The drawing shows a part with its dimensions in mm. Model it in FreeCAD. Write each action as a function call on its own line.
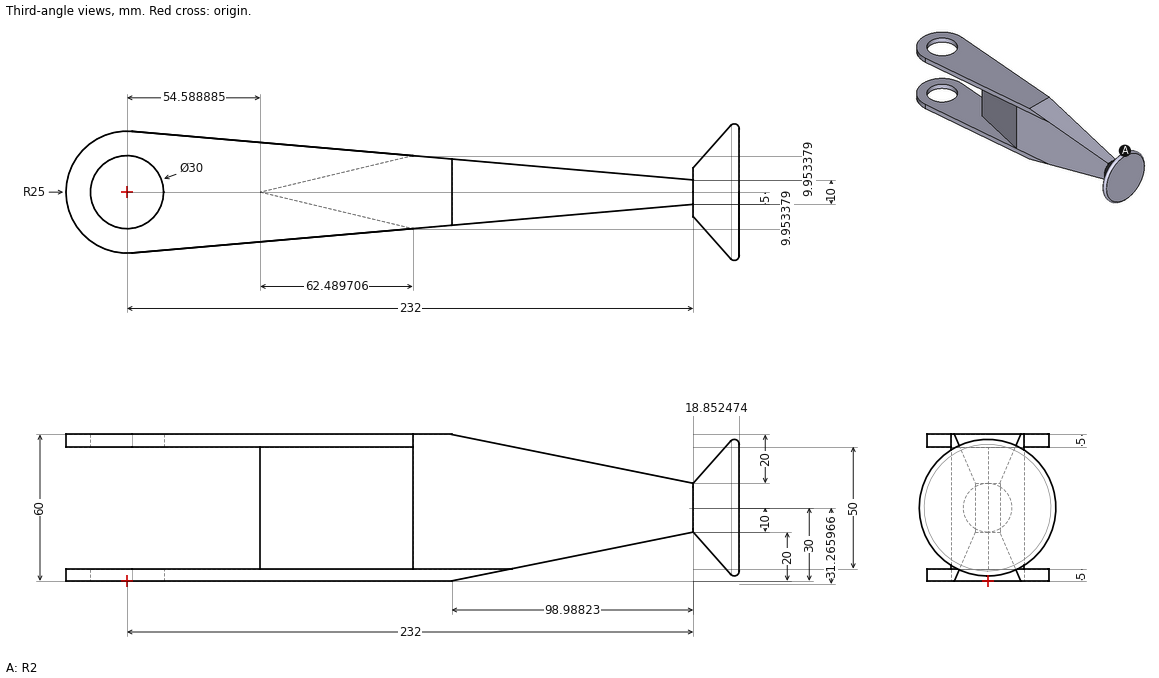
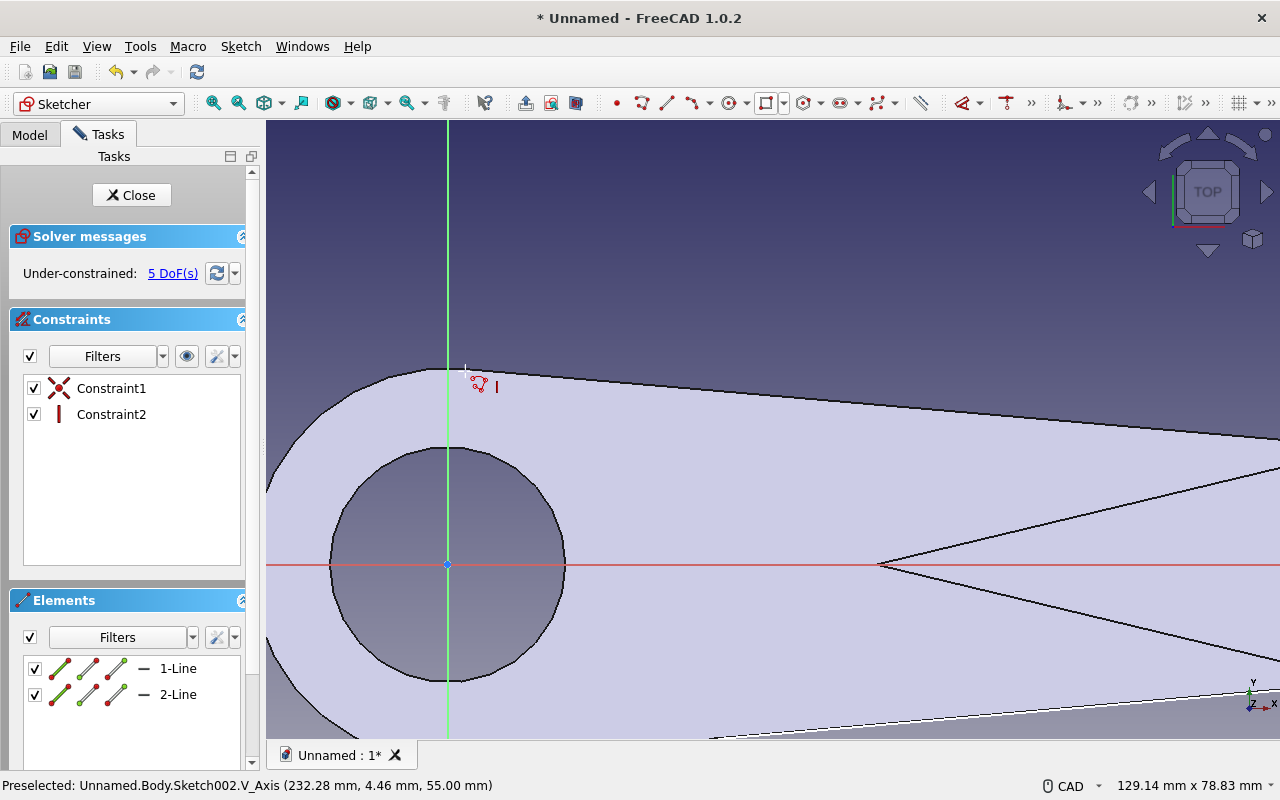
click(465, 369)
right_click(465, 369)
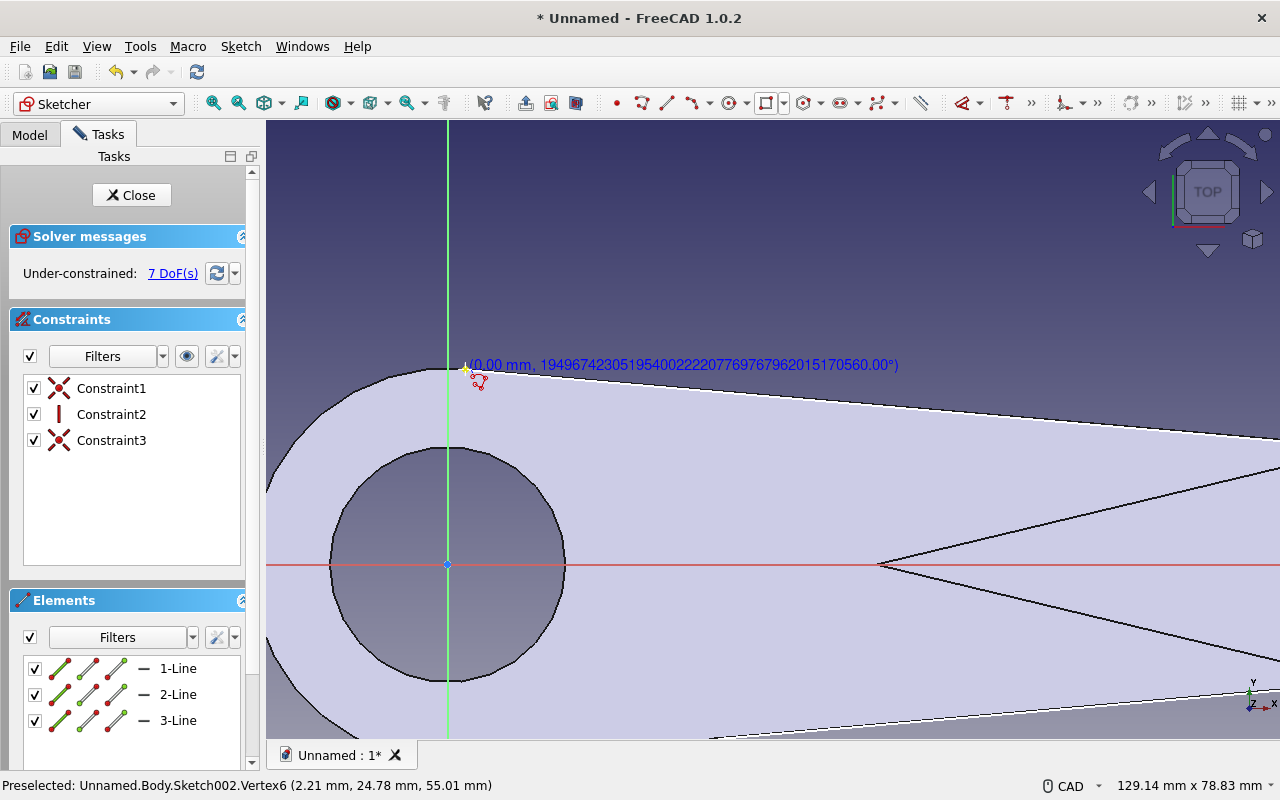
click(692, 104)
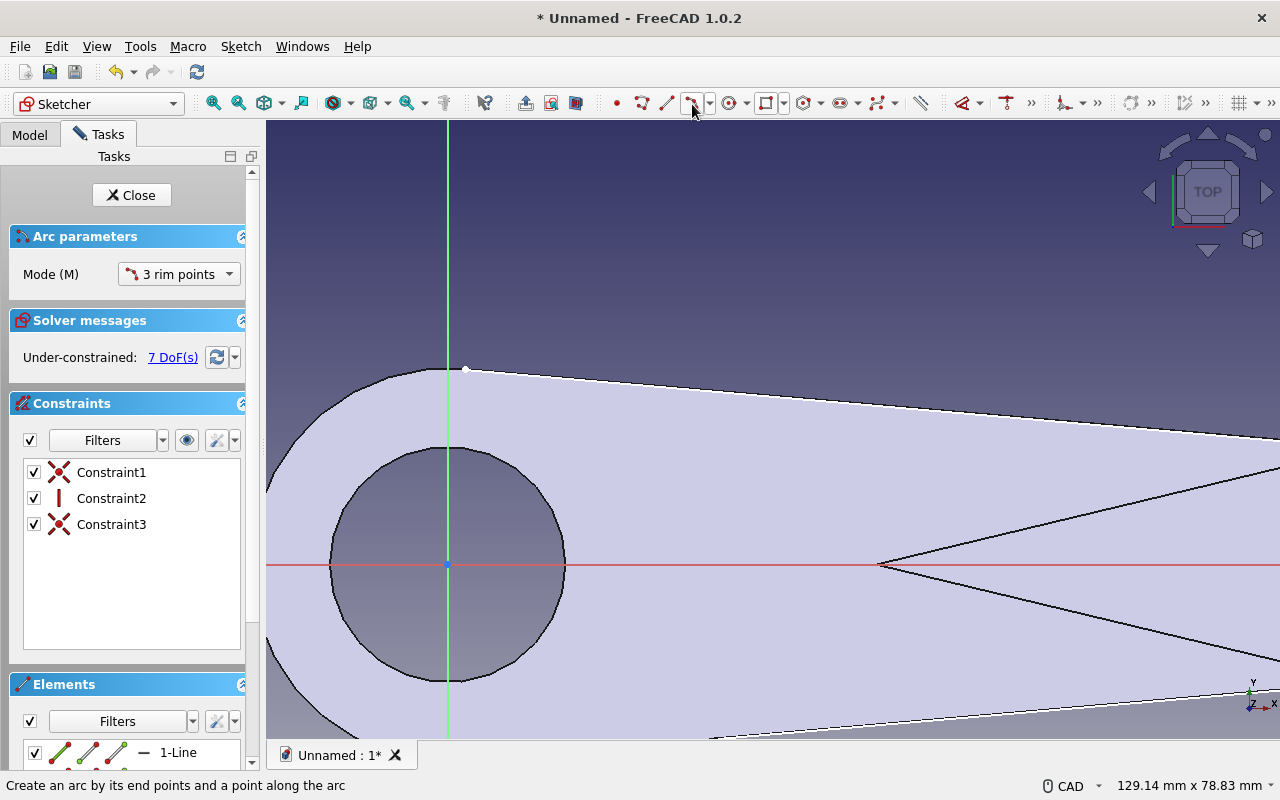
click(465, 370)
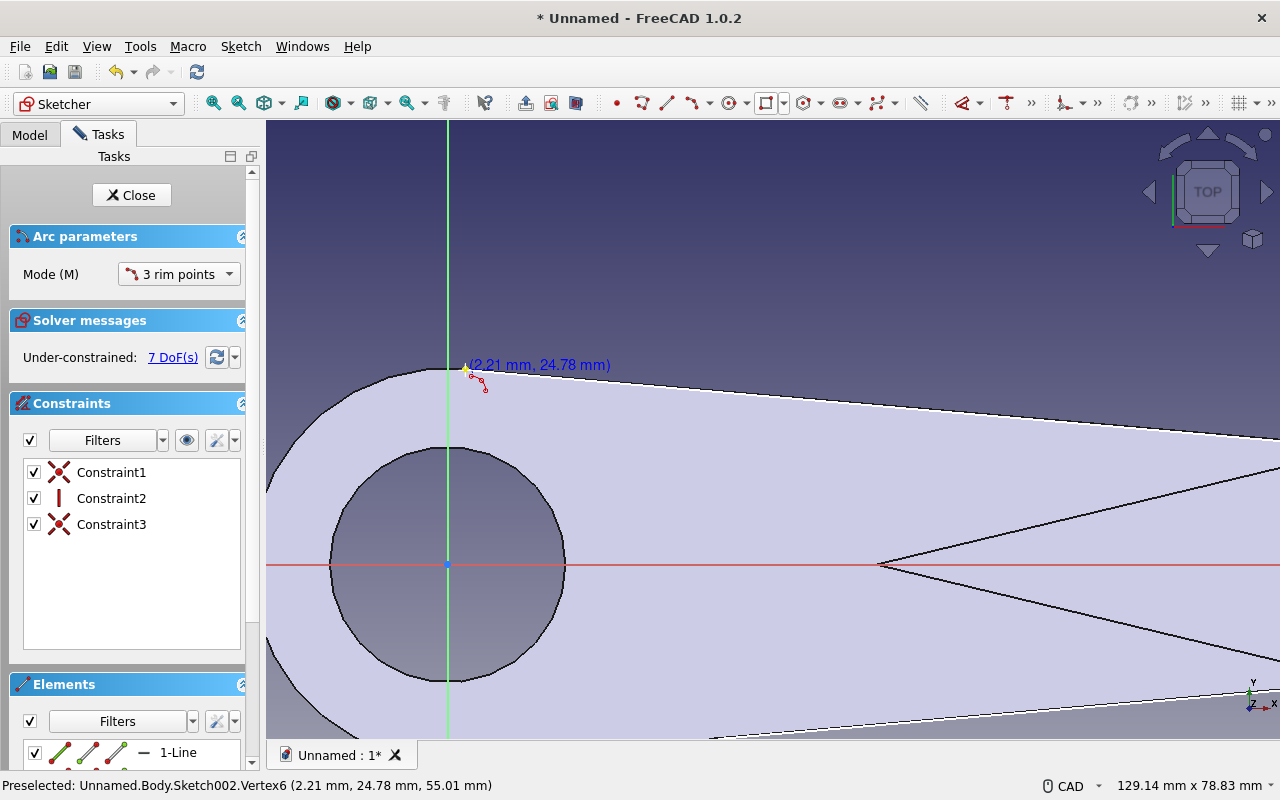
scroll(465, 371, down, 6)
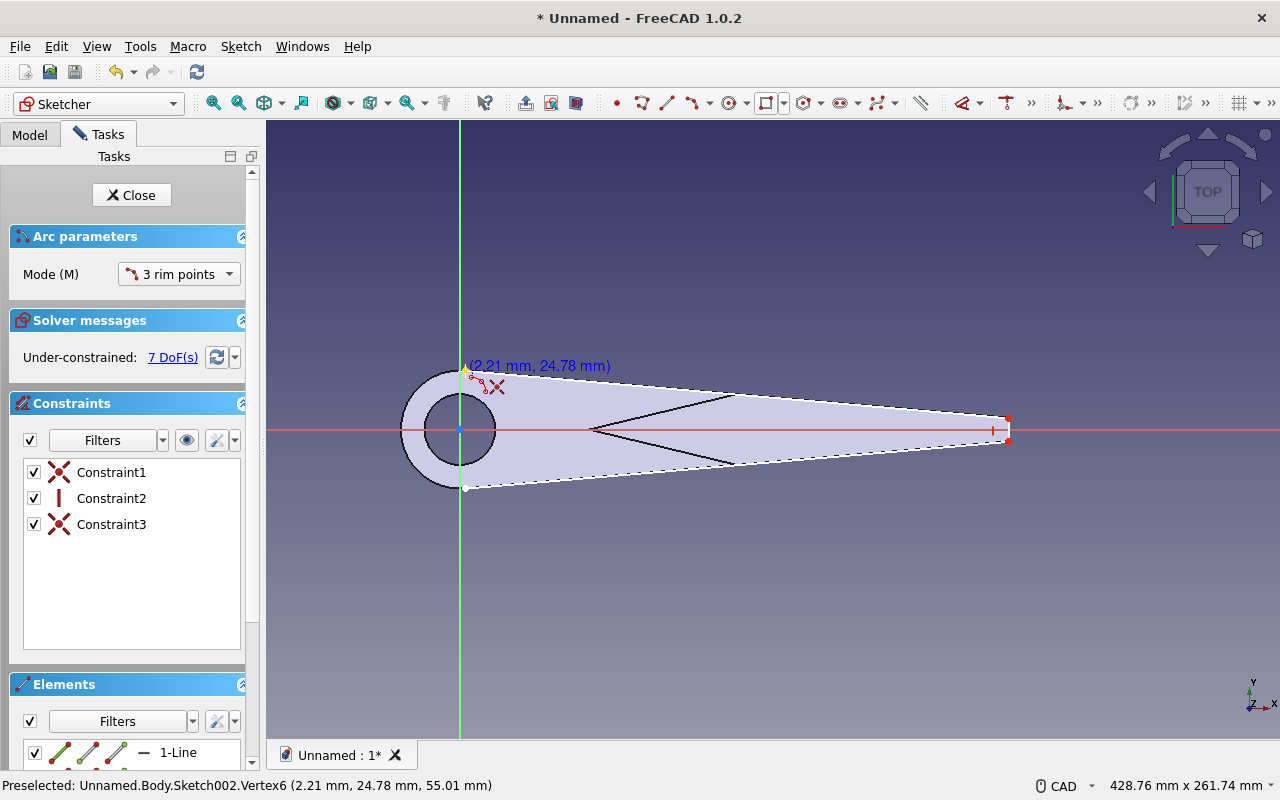
scroll(465, 488, up, 6)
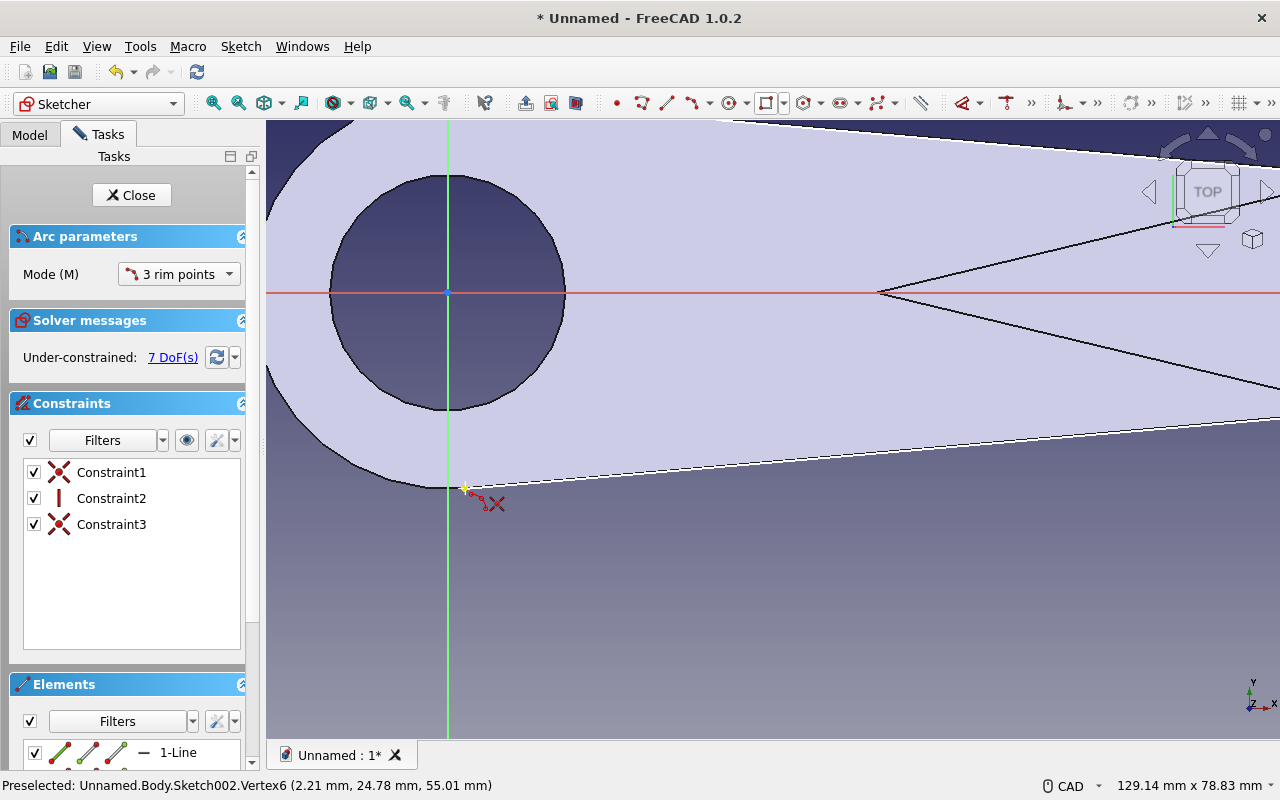
click(465, 489)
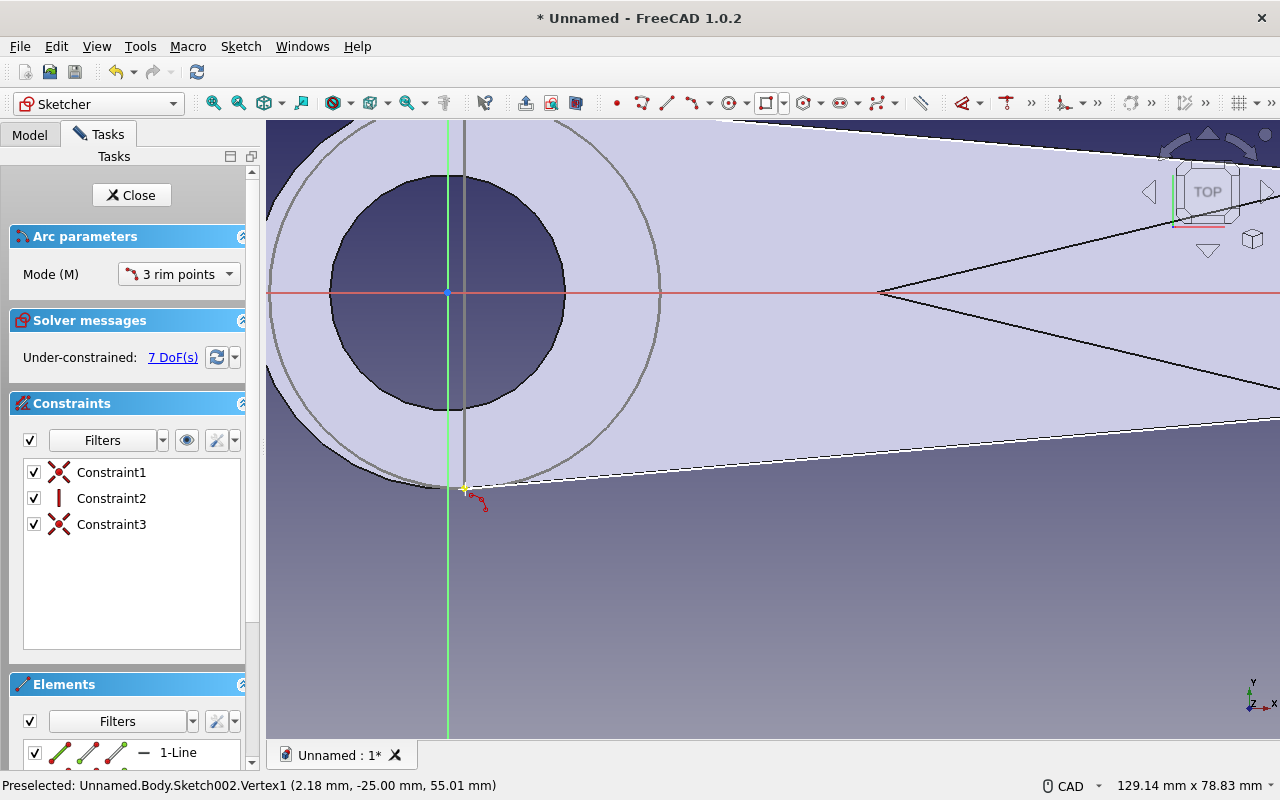
scroll(465, 488, down, 6)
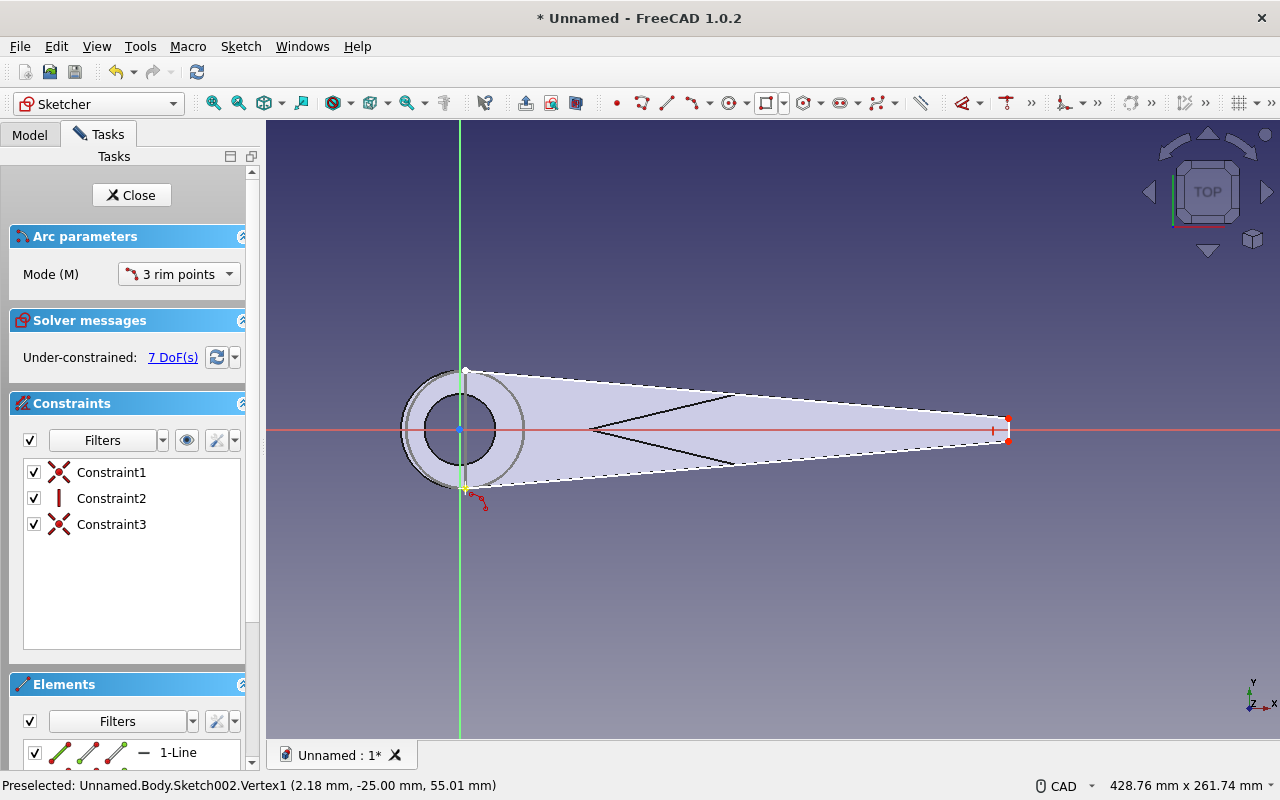
click(404, 410)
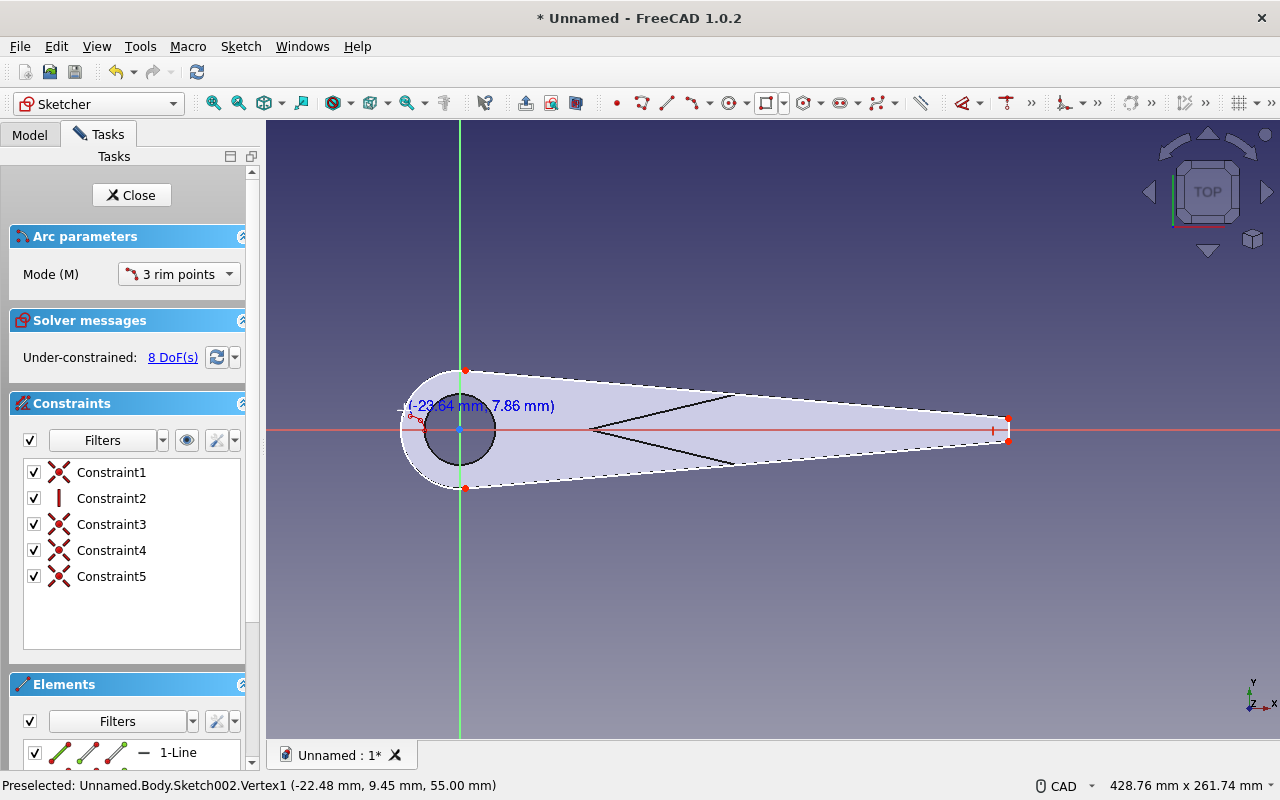
click(728, 104)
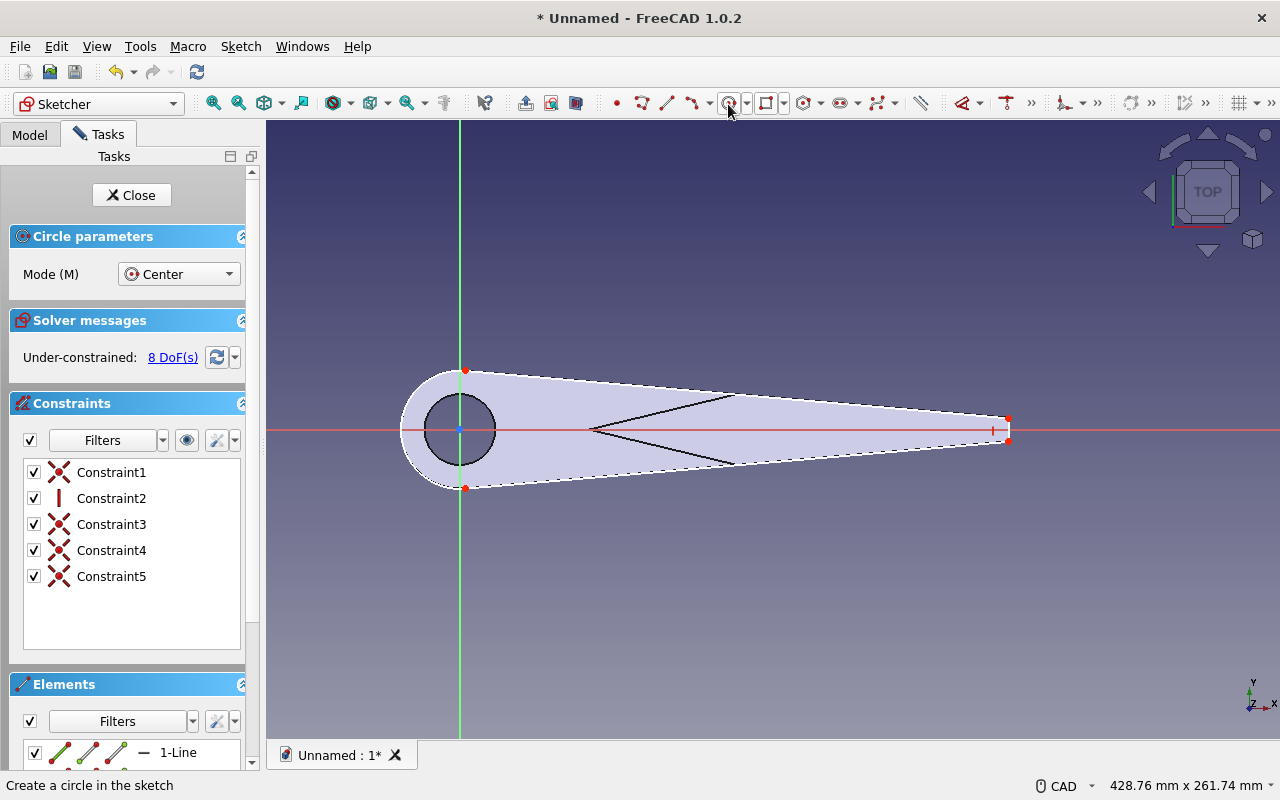
click(460, 430)
click(485, 405)
key(Escape)